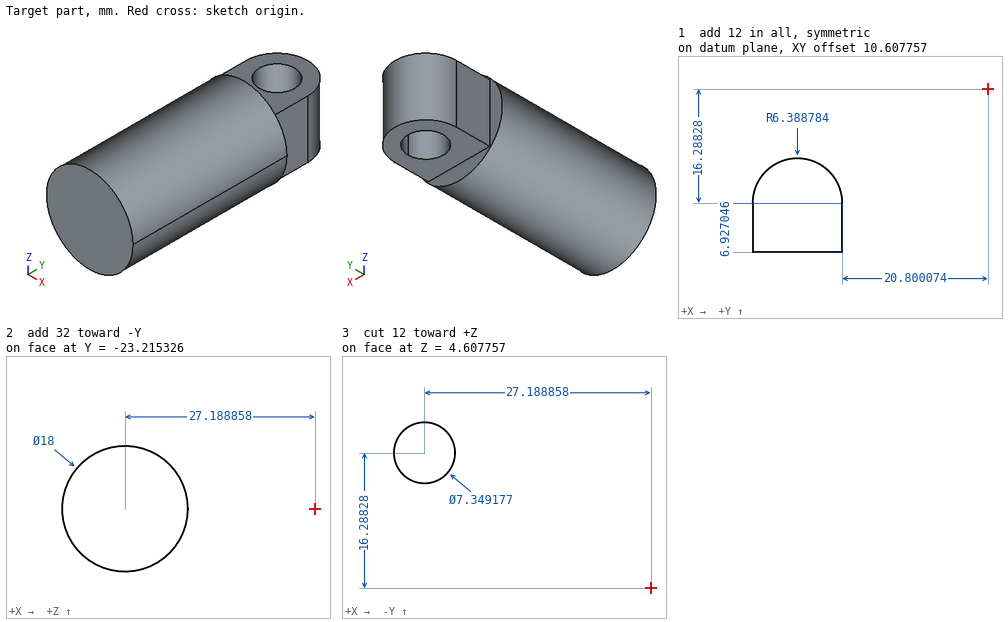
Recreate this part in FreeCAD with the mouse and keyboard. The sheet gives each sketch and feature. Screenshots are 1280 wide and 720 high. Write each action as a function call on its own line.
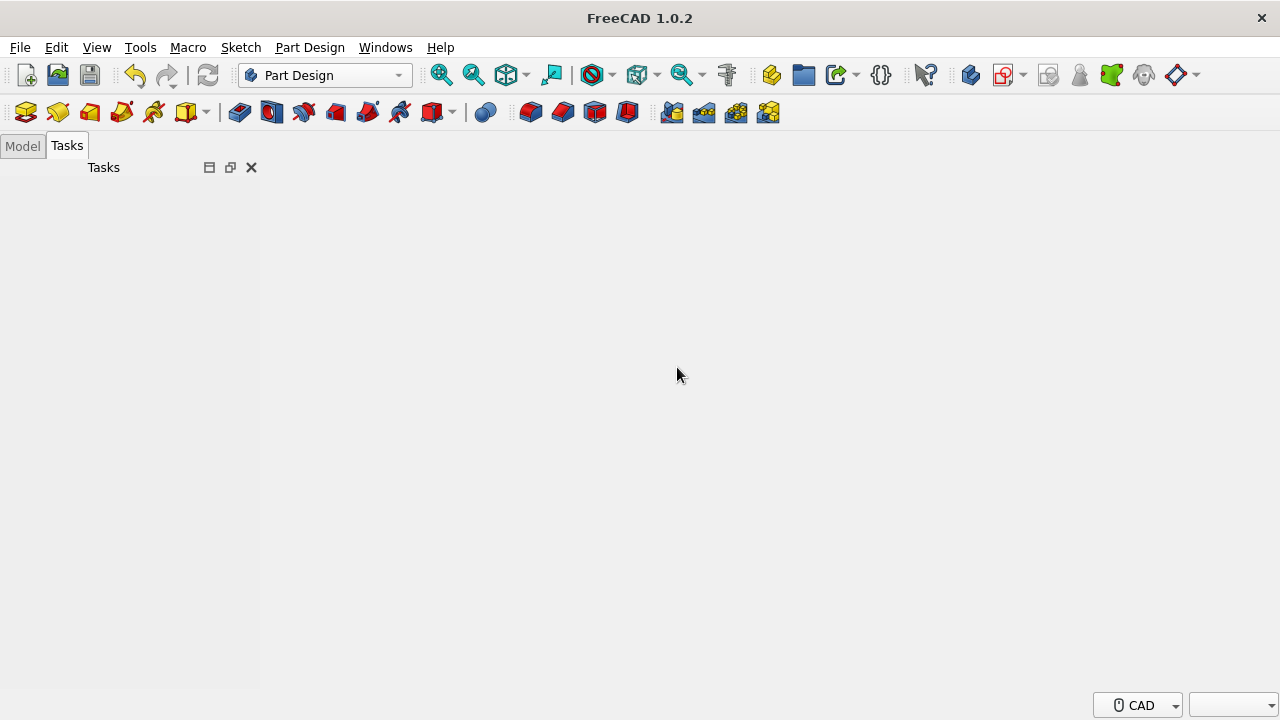
click(26, 76)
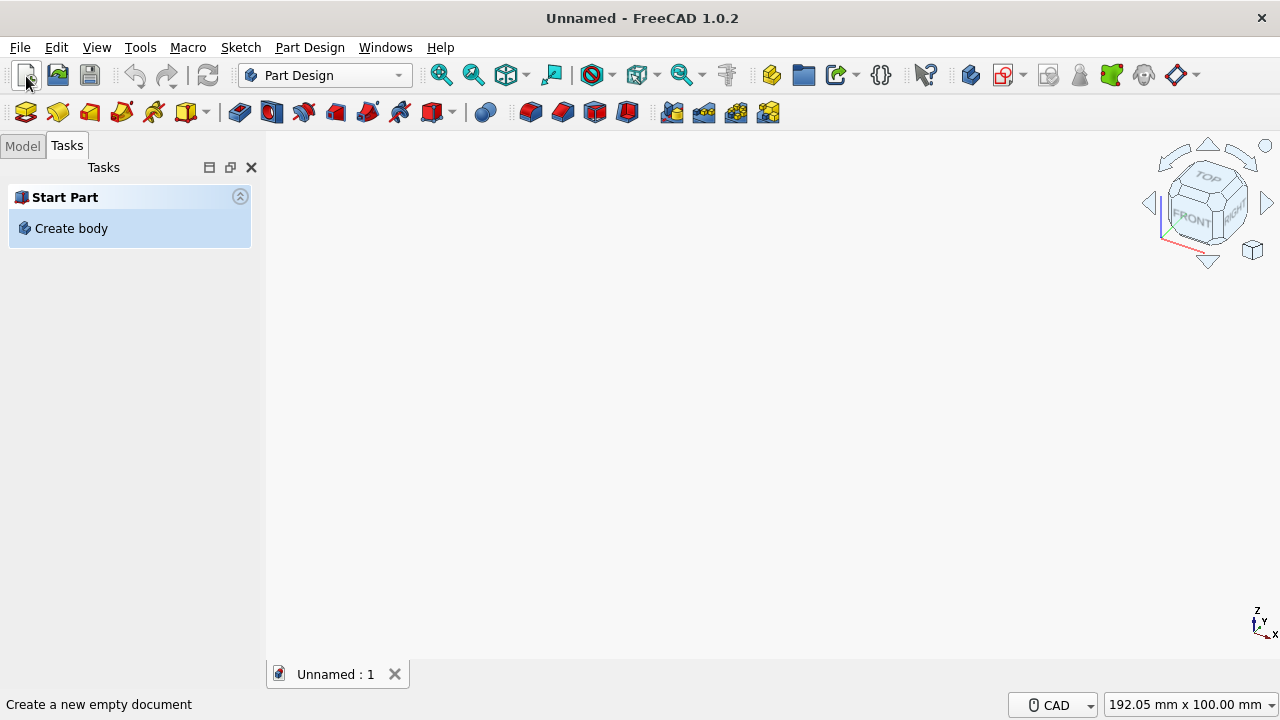
click(972, 76)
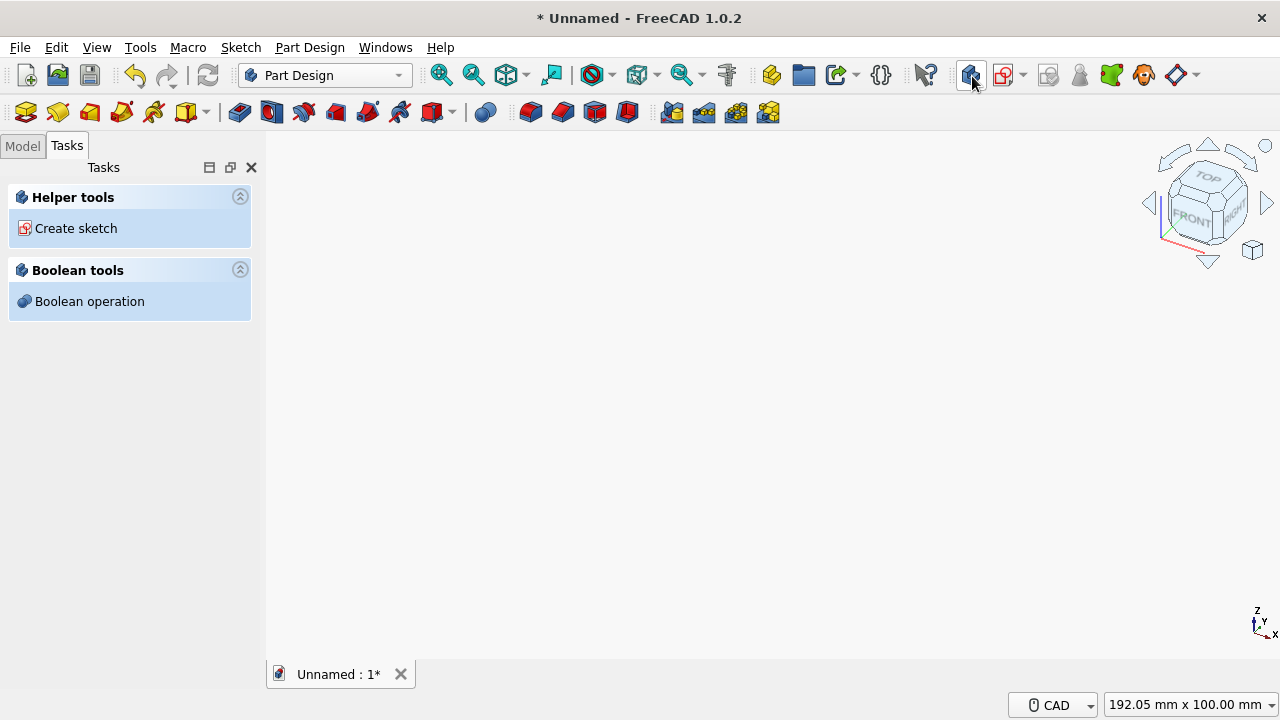
click(23, 145)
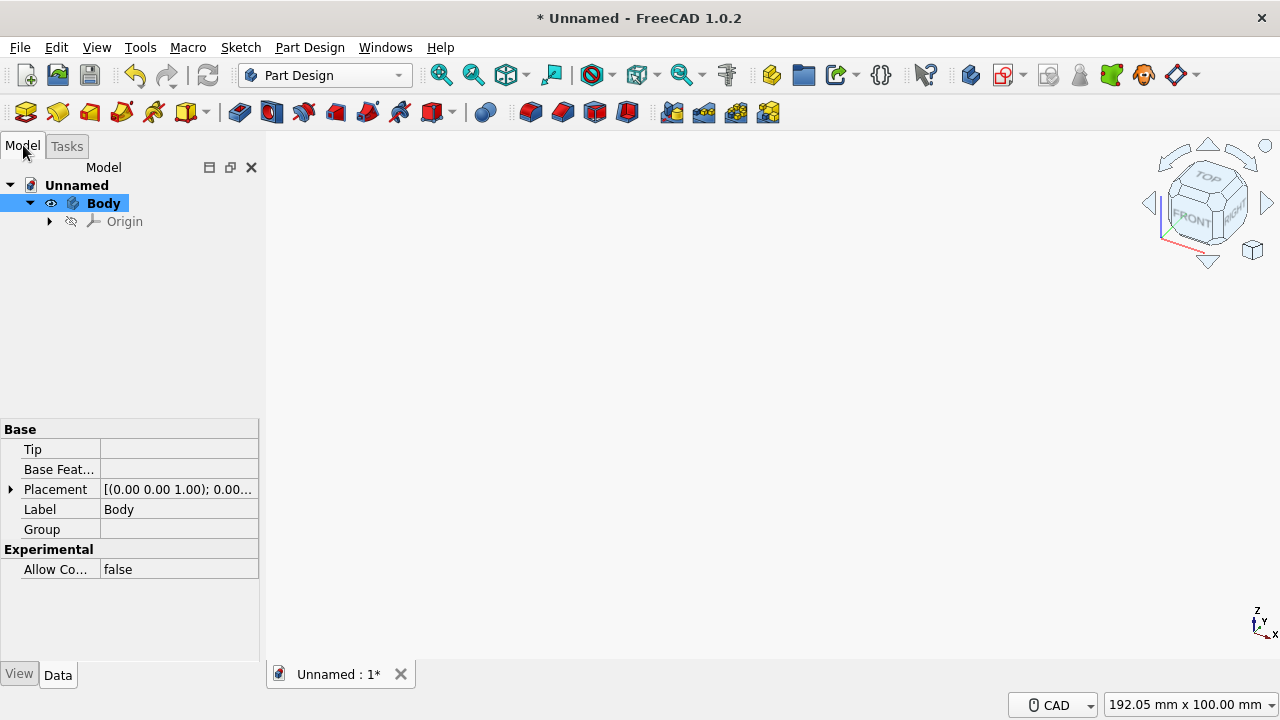
click(50, 221)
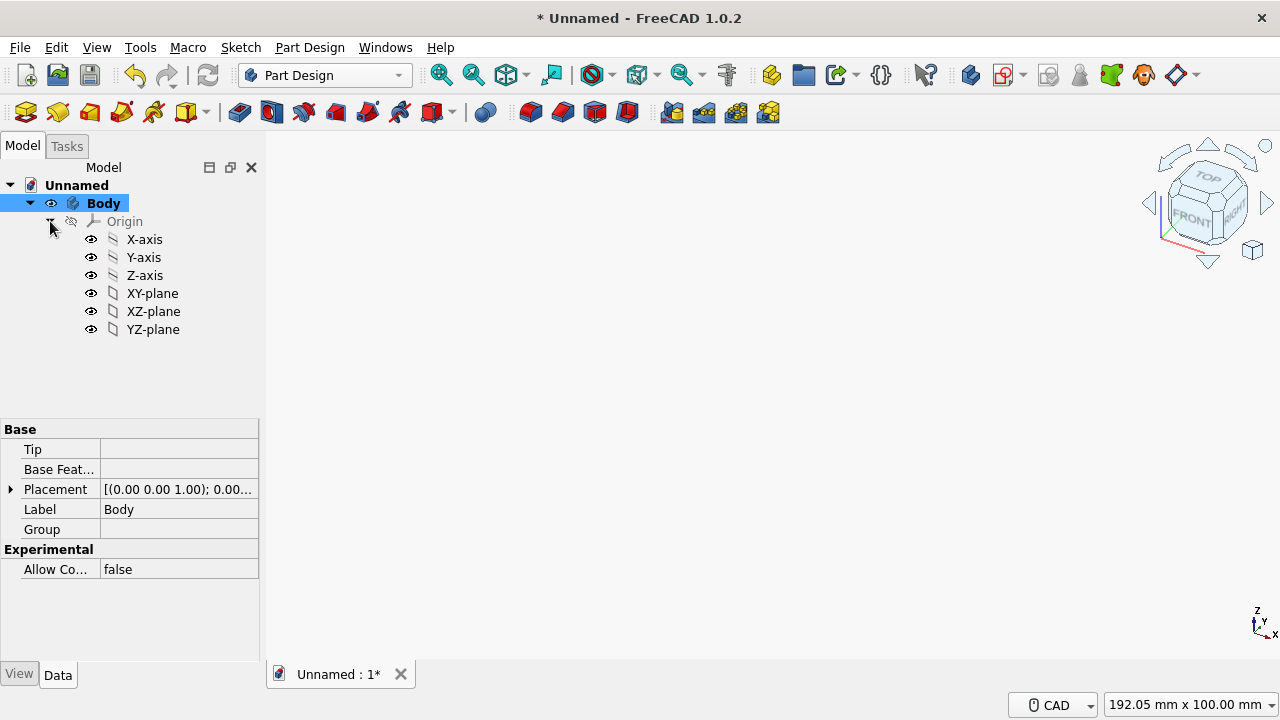
click(136, 293)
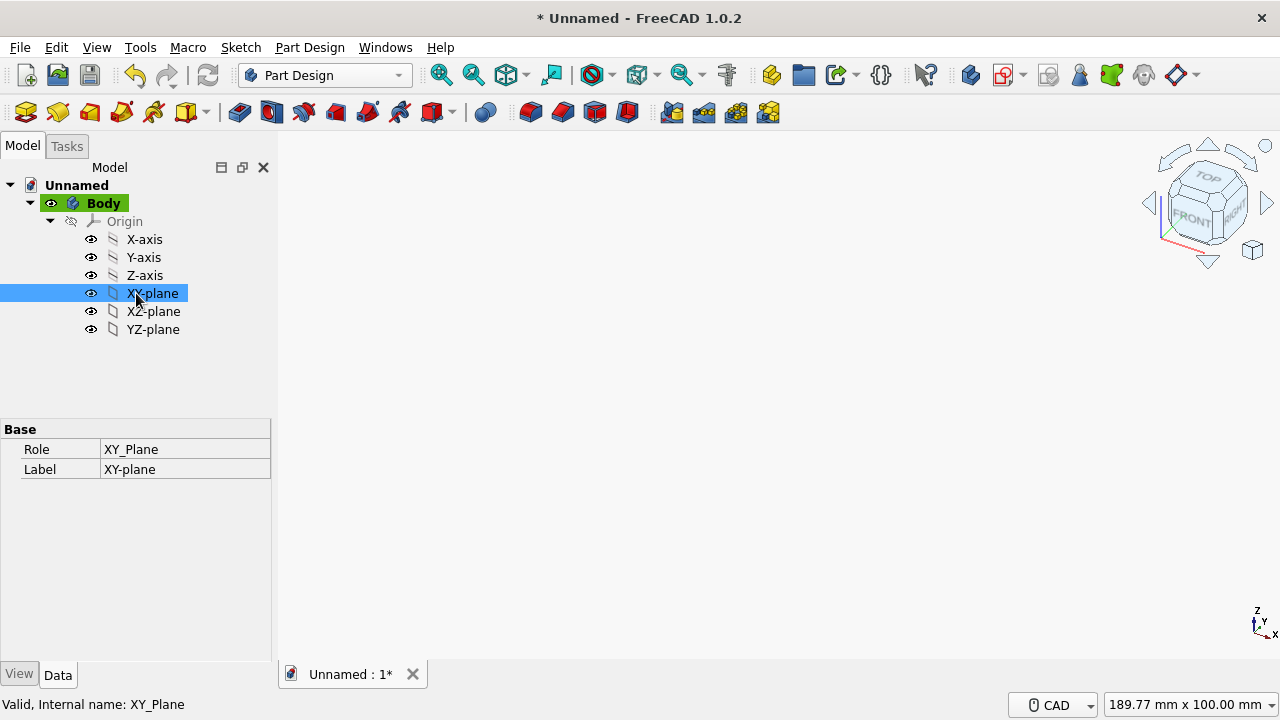
click(1176, 76)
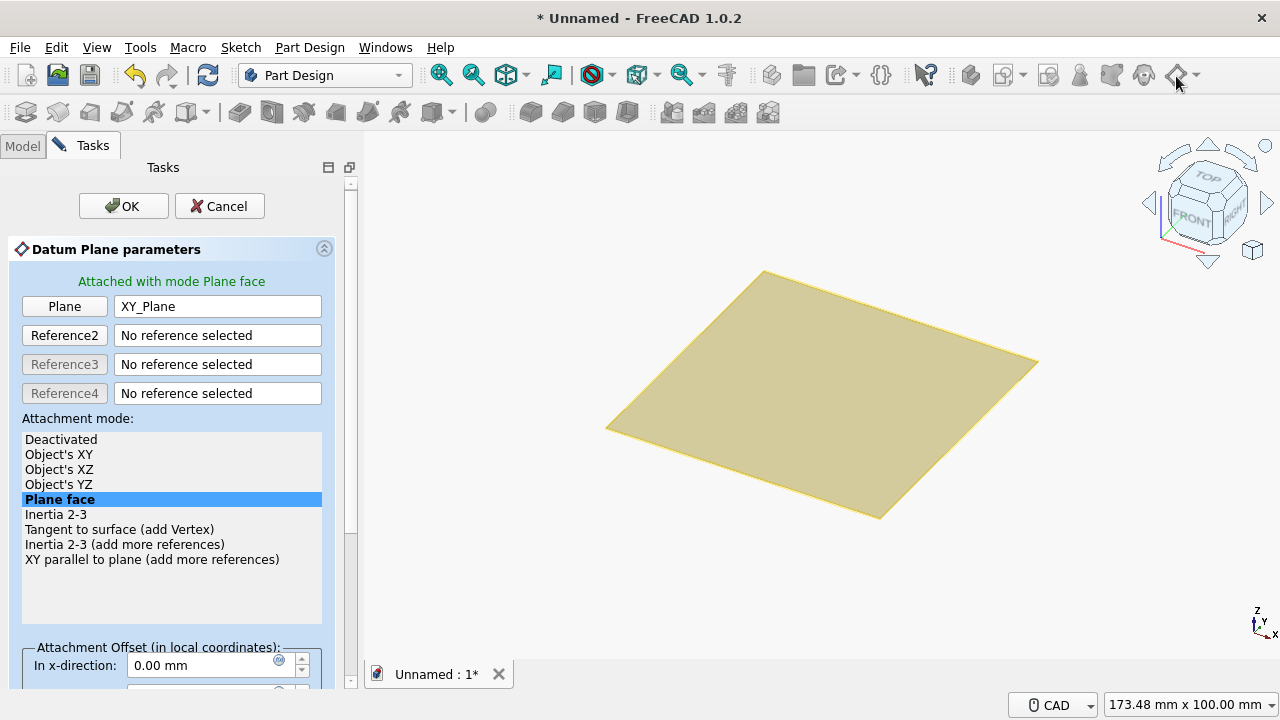
scroll(351, 432, down, 2)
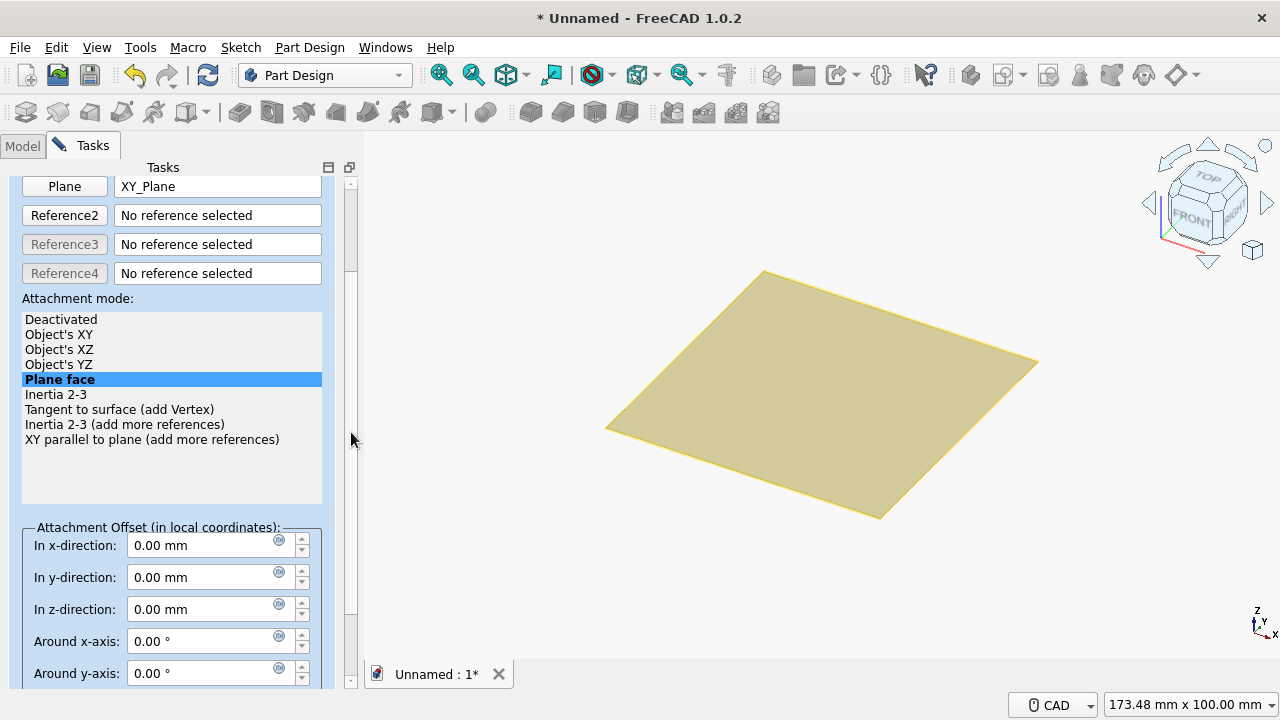
triple_click(210, 609)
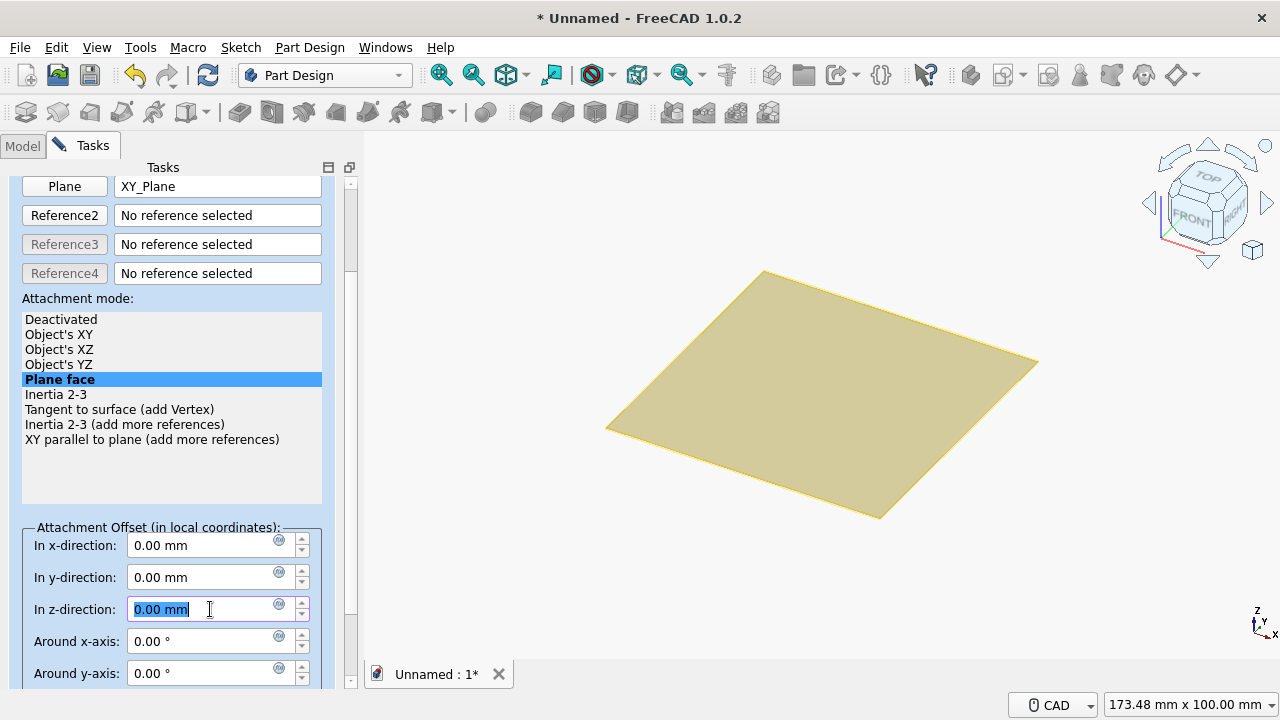
text(10.607757)
key(Tab)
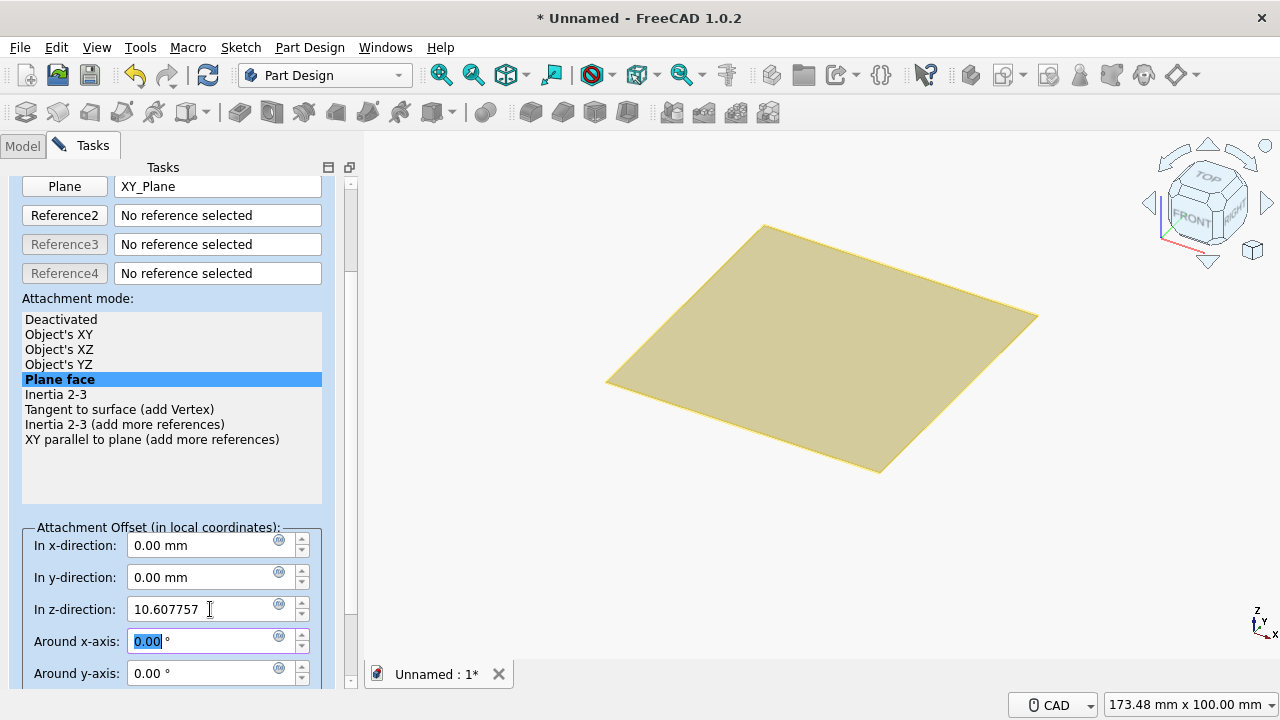
scroll(351, 432, up, 3)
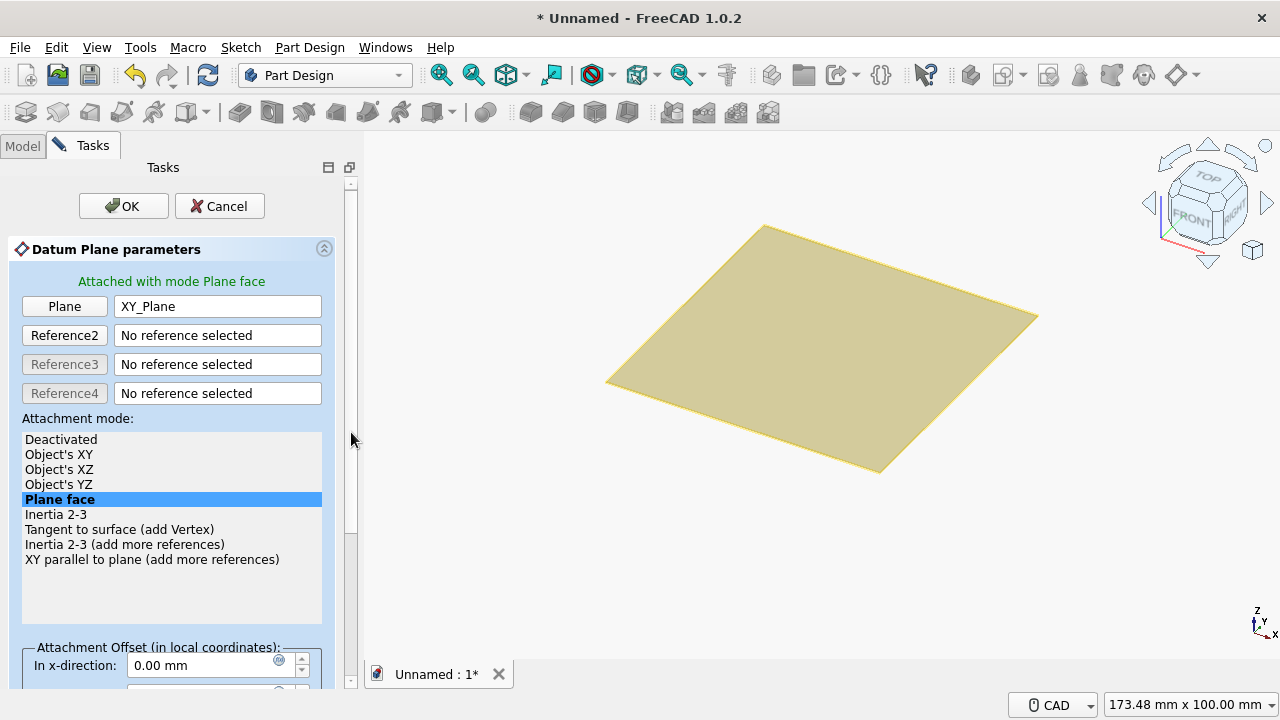
click(124, 206)